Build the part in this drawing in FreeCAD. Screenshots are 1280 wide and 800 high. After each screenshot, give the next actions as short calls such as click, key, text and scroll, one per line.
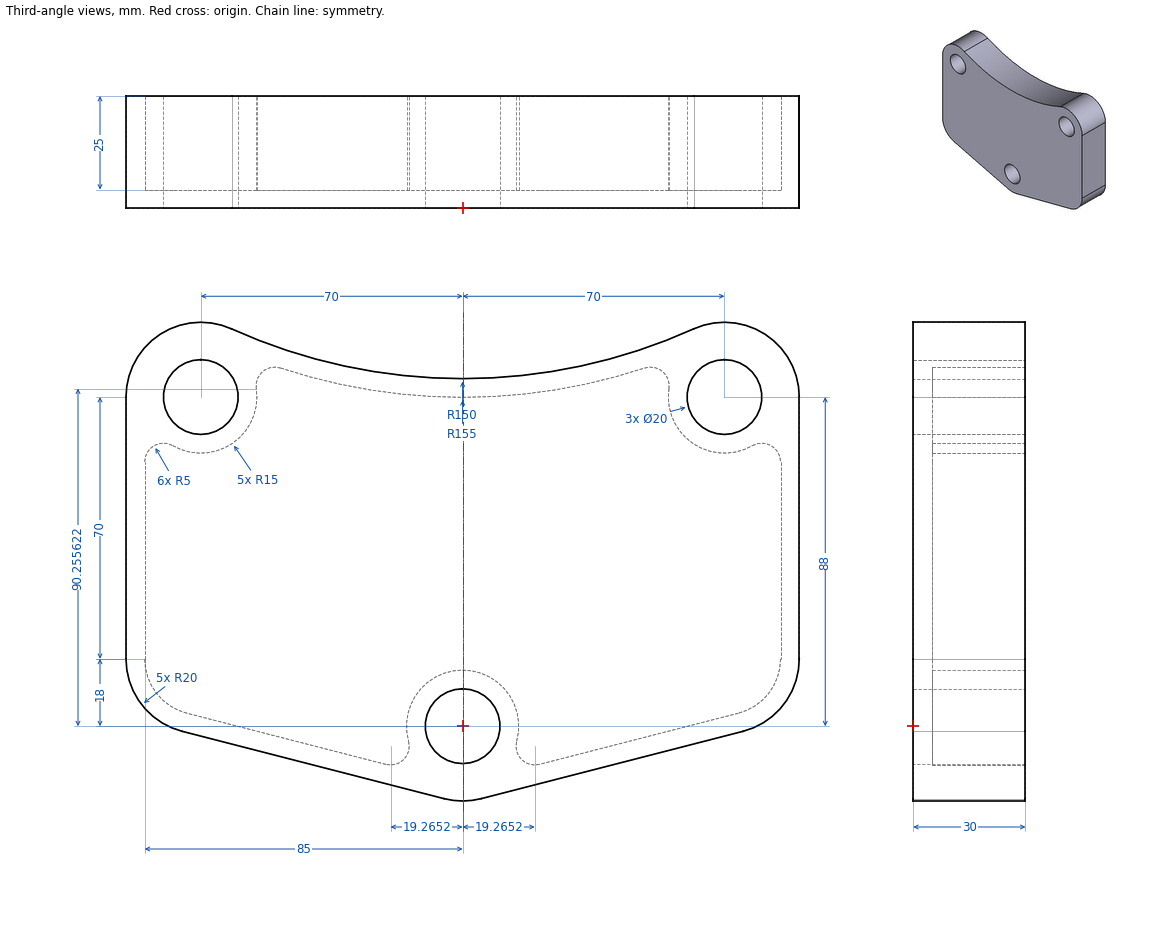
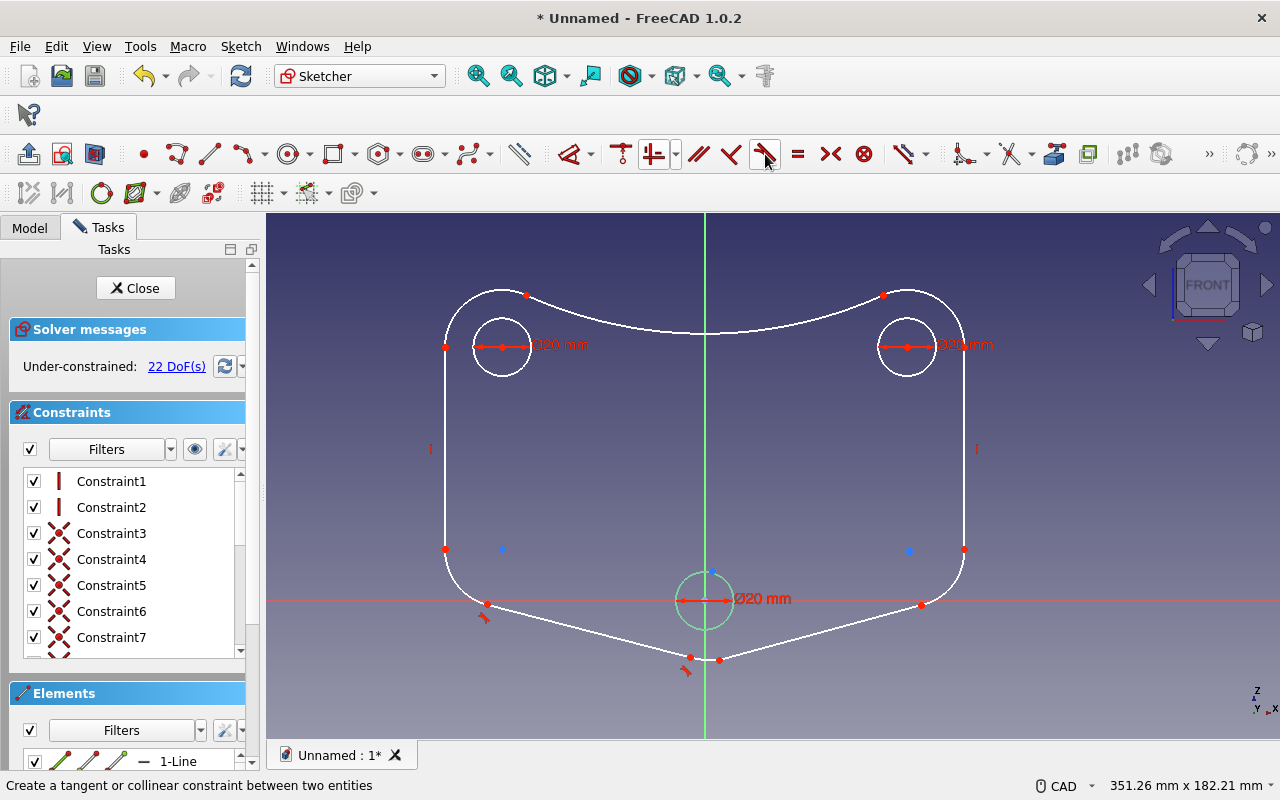
click(445, 489)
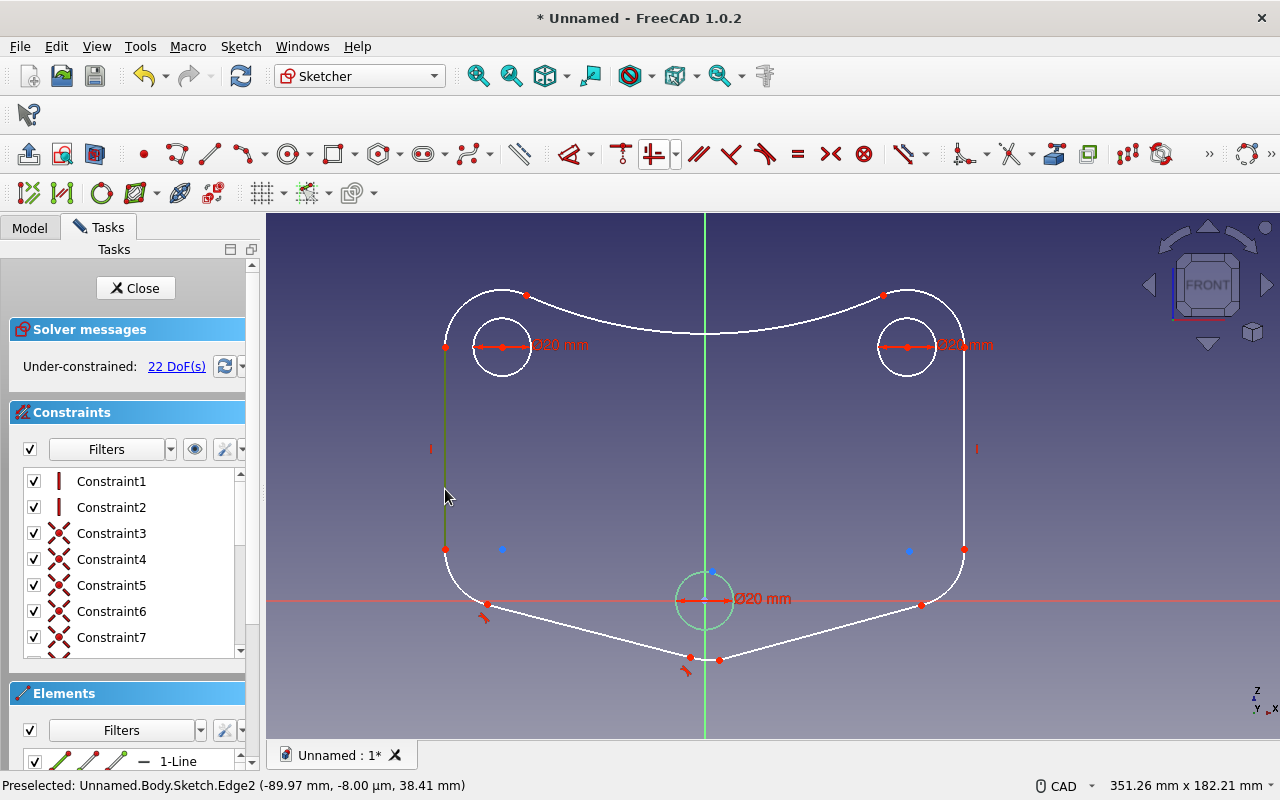
click(449, 572)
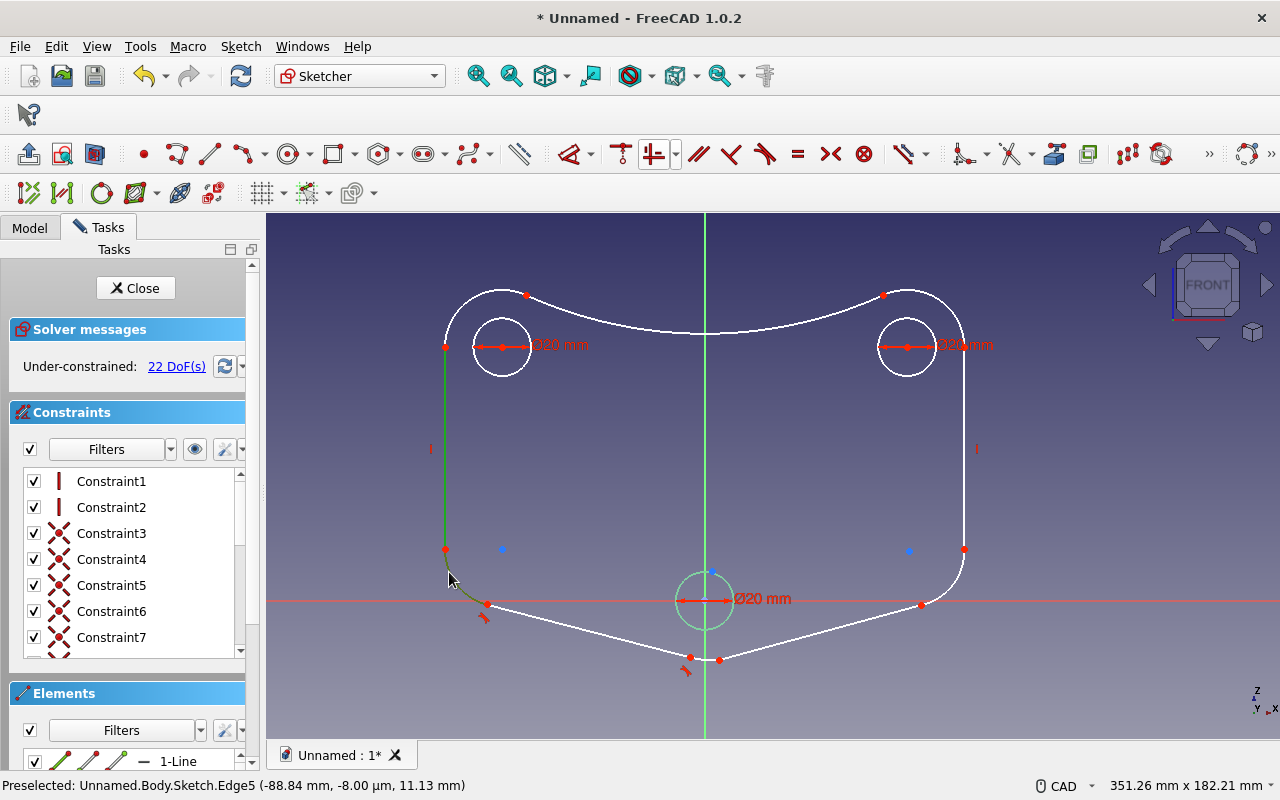
click(765, 154)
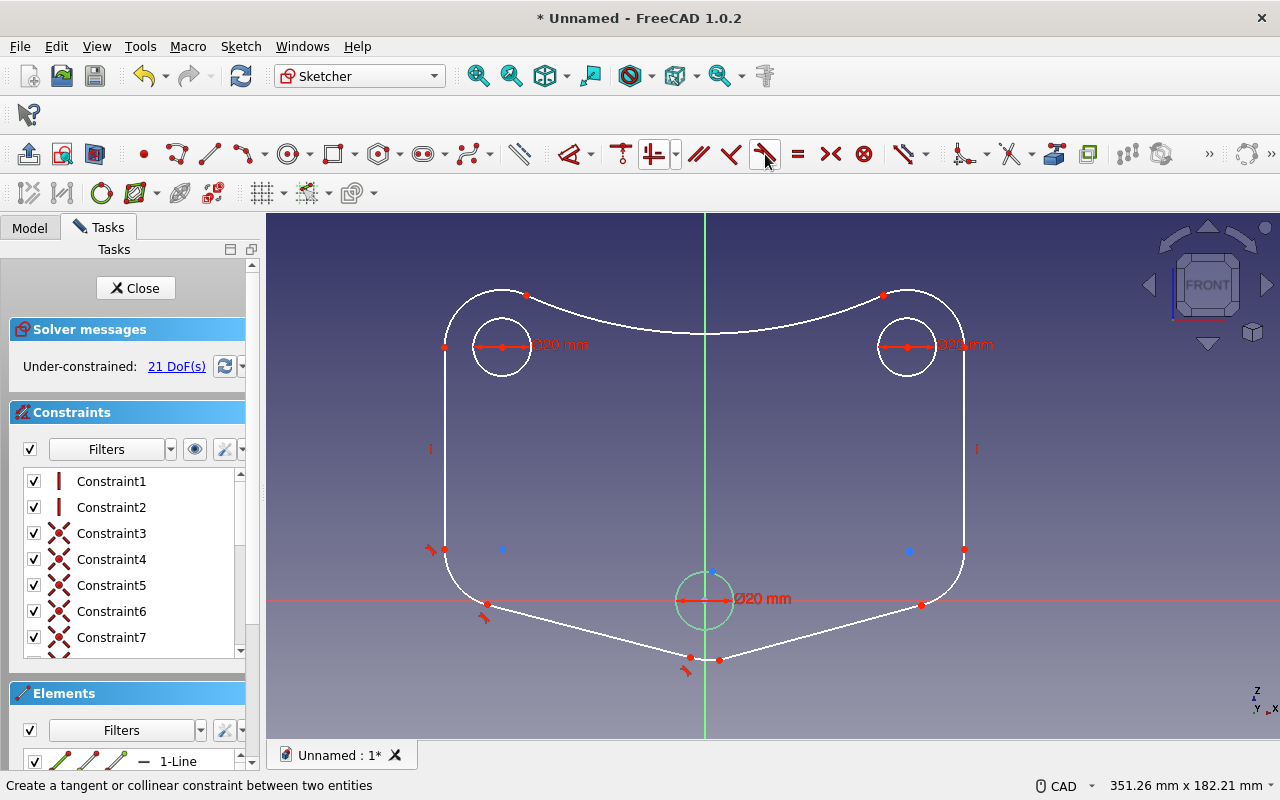
click(445, 489)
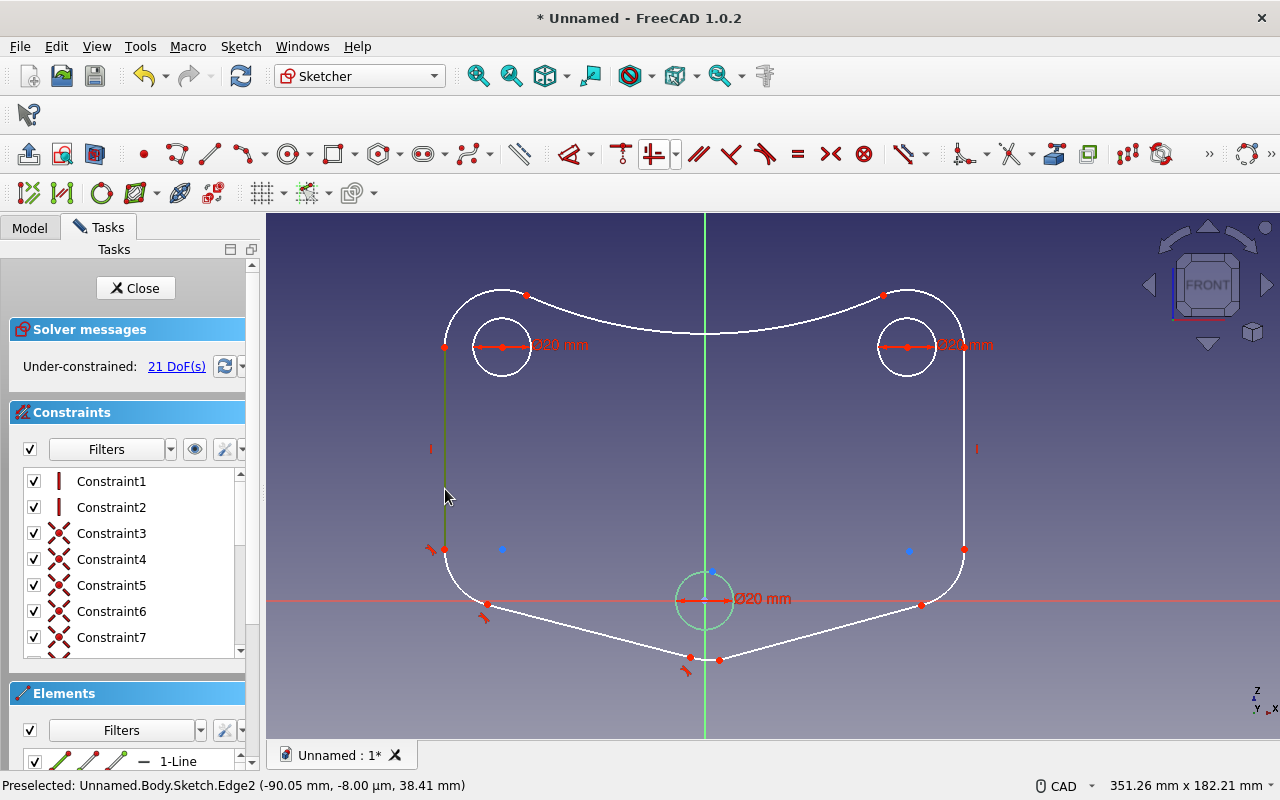
click(492, 291)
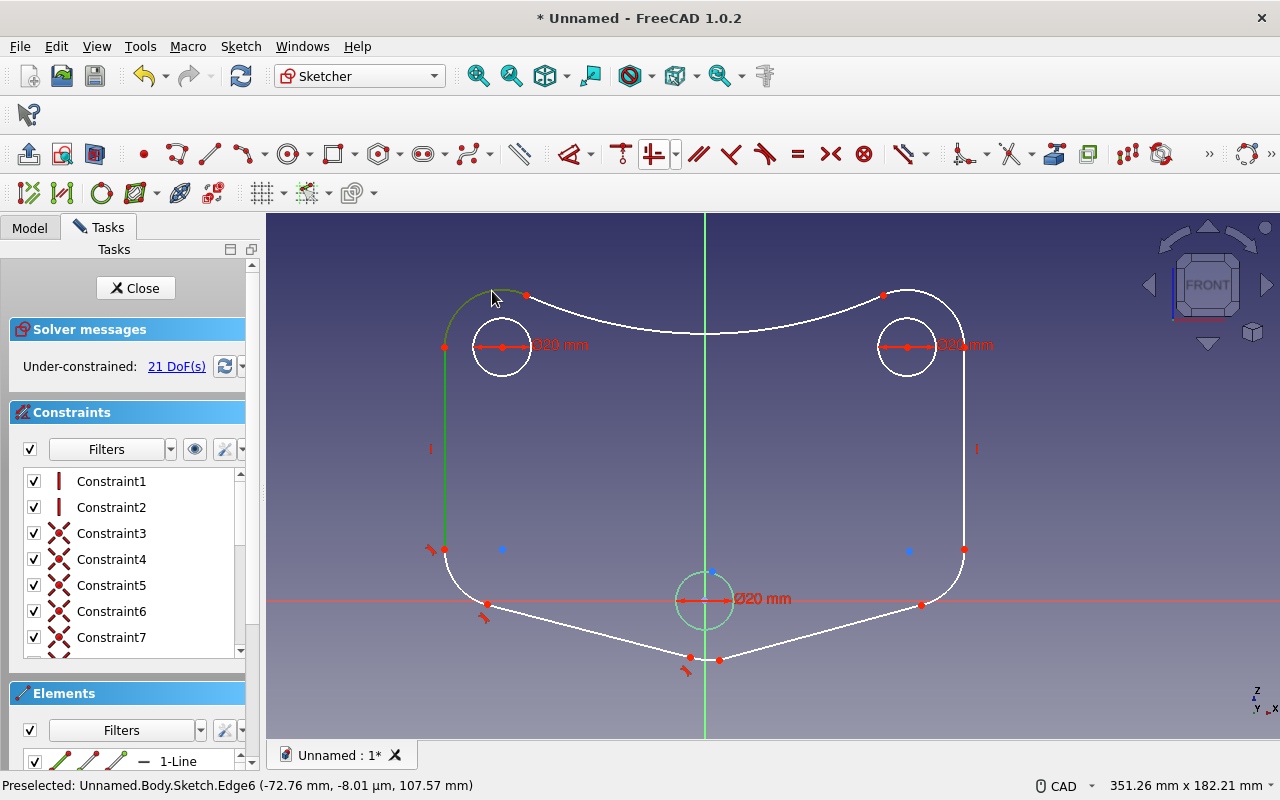
click(765, 154)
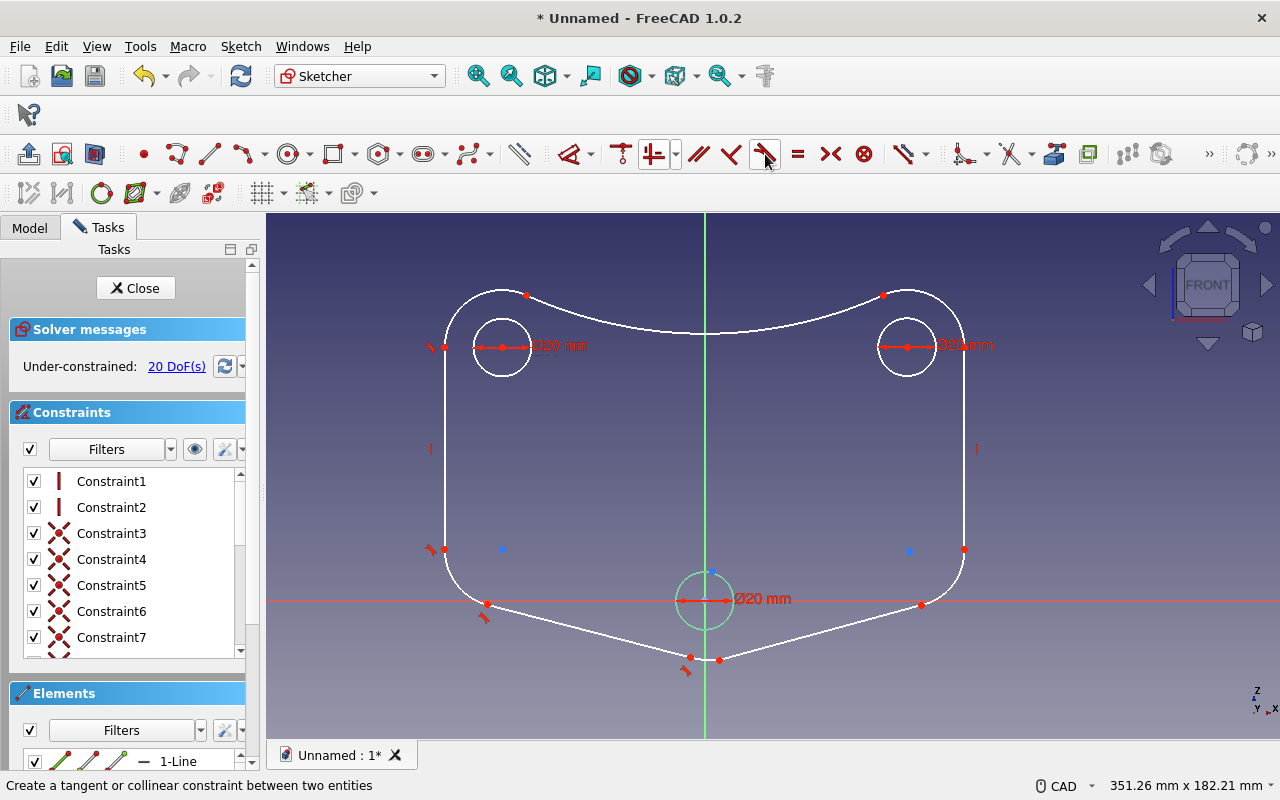
click(964, 408)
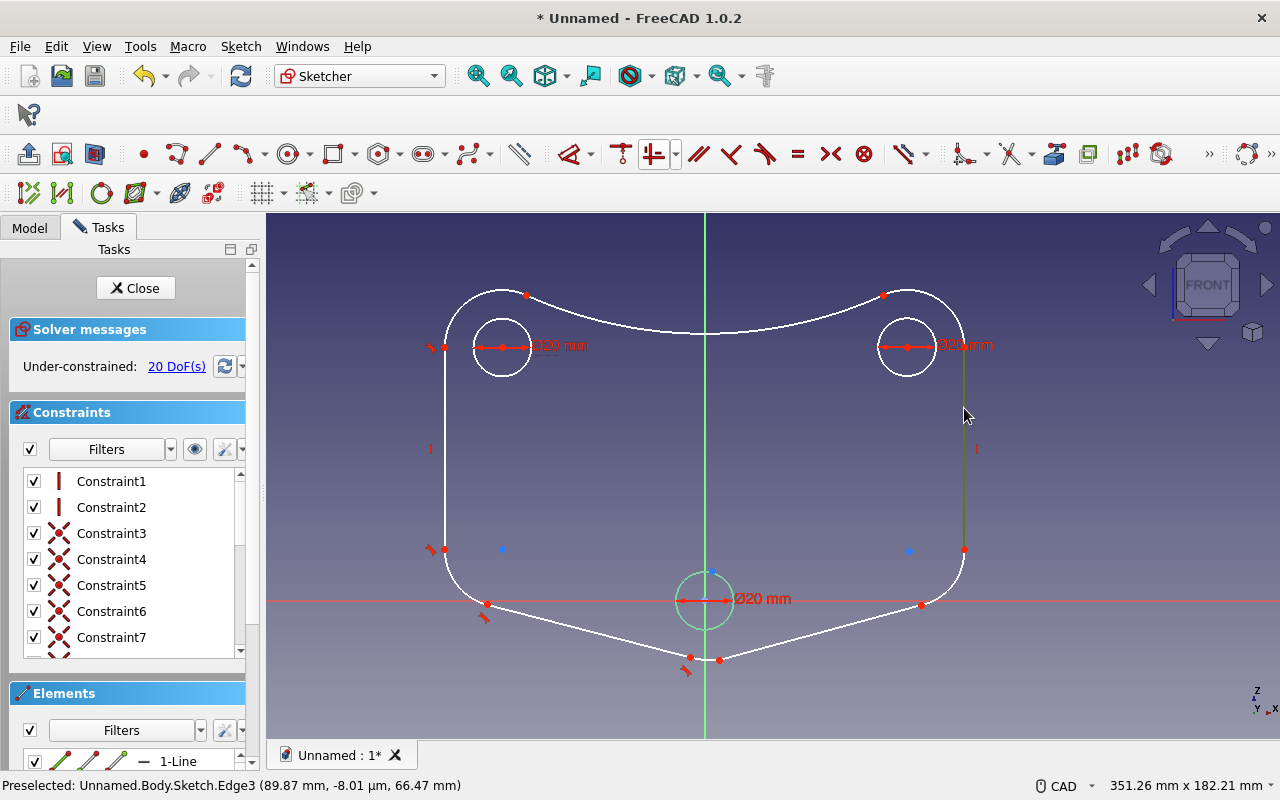
click(954, 315)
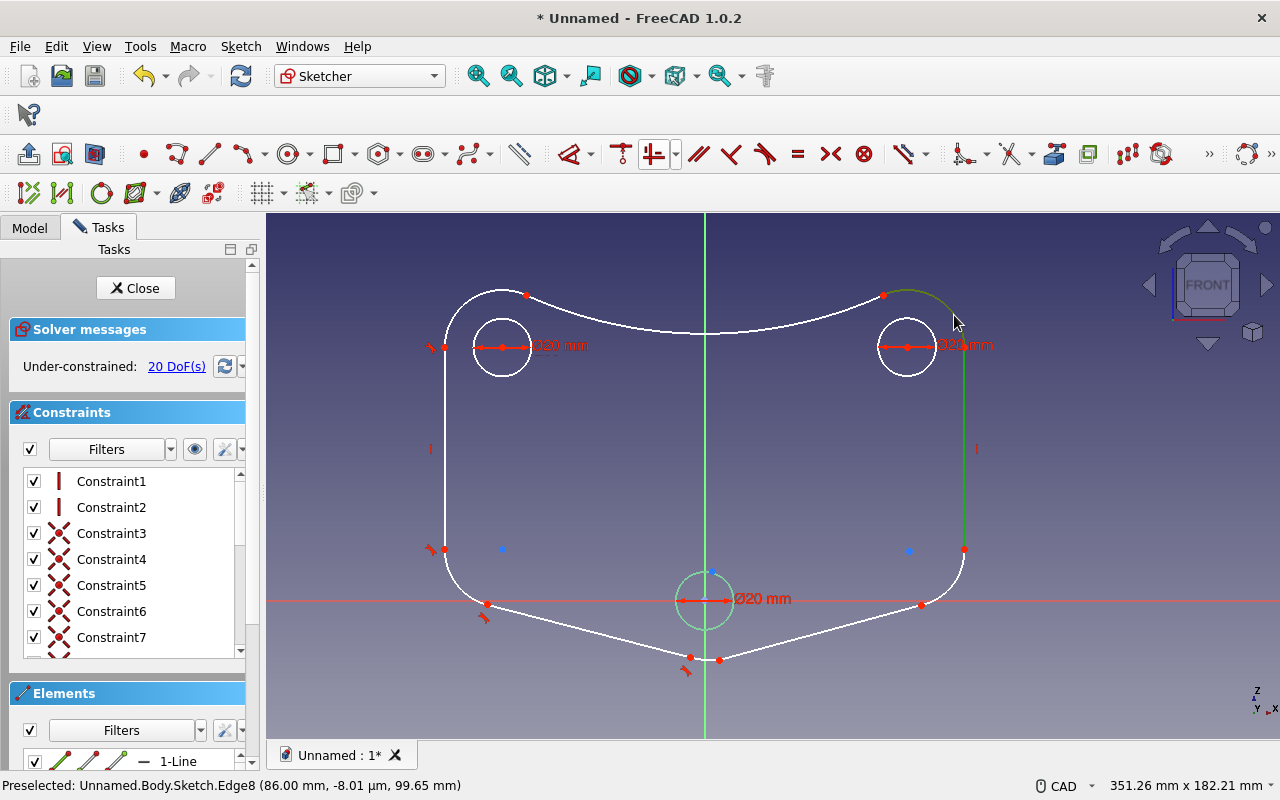
click(765, 154)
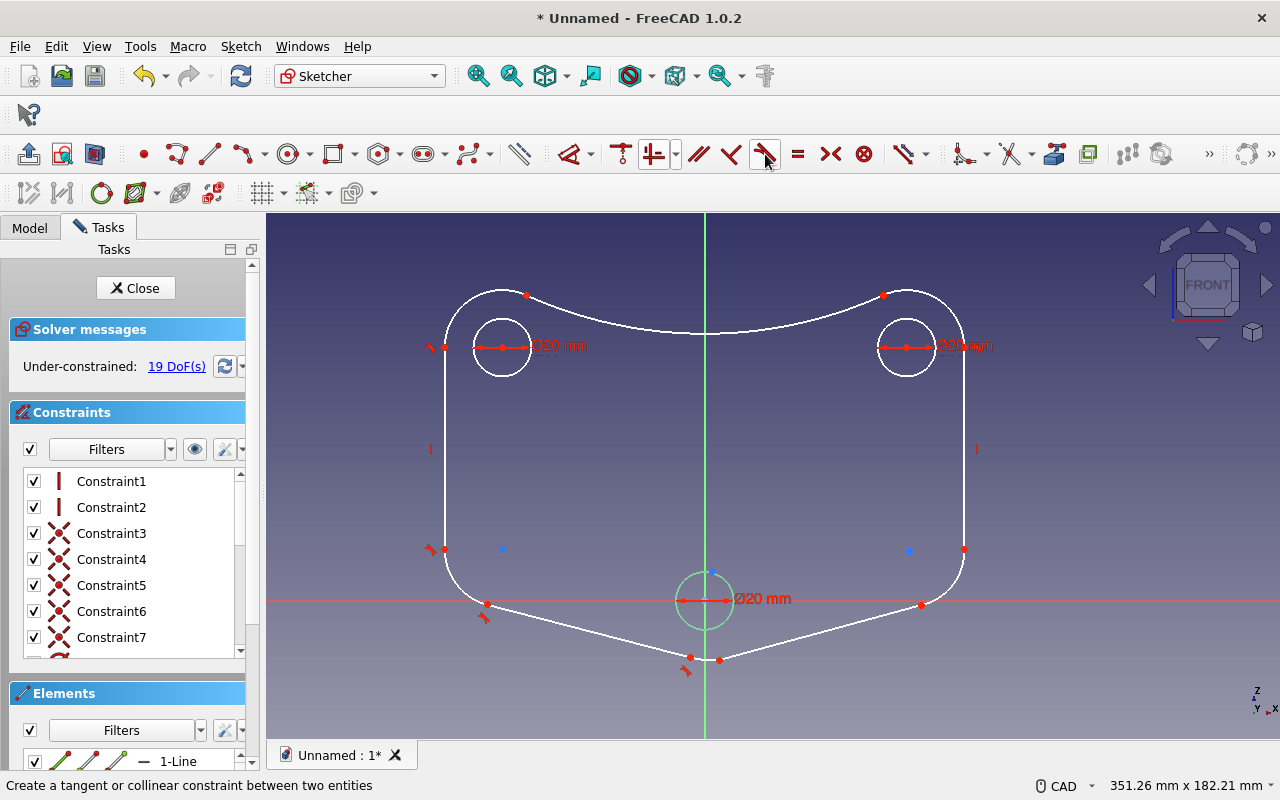
click(964, 408)